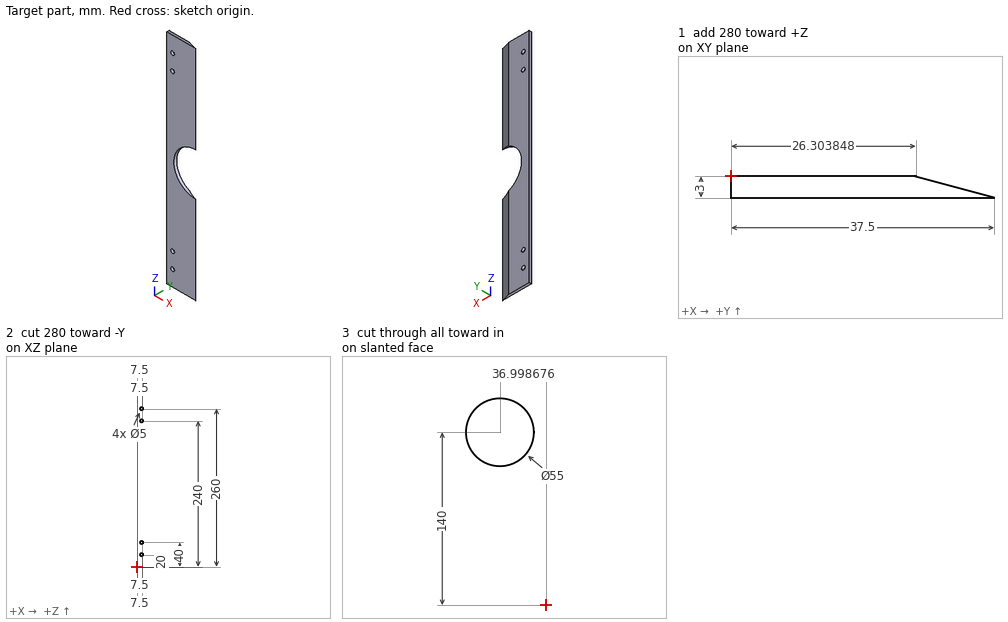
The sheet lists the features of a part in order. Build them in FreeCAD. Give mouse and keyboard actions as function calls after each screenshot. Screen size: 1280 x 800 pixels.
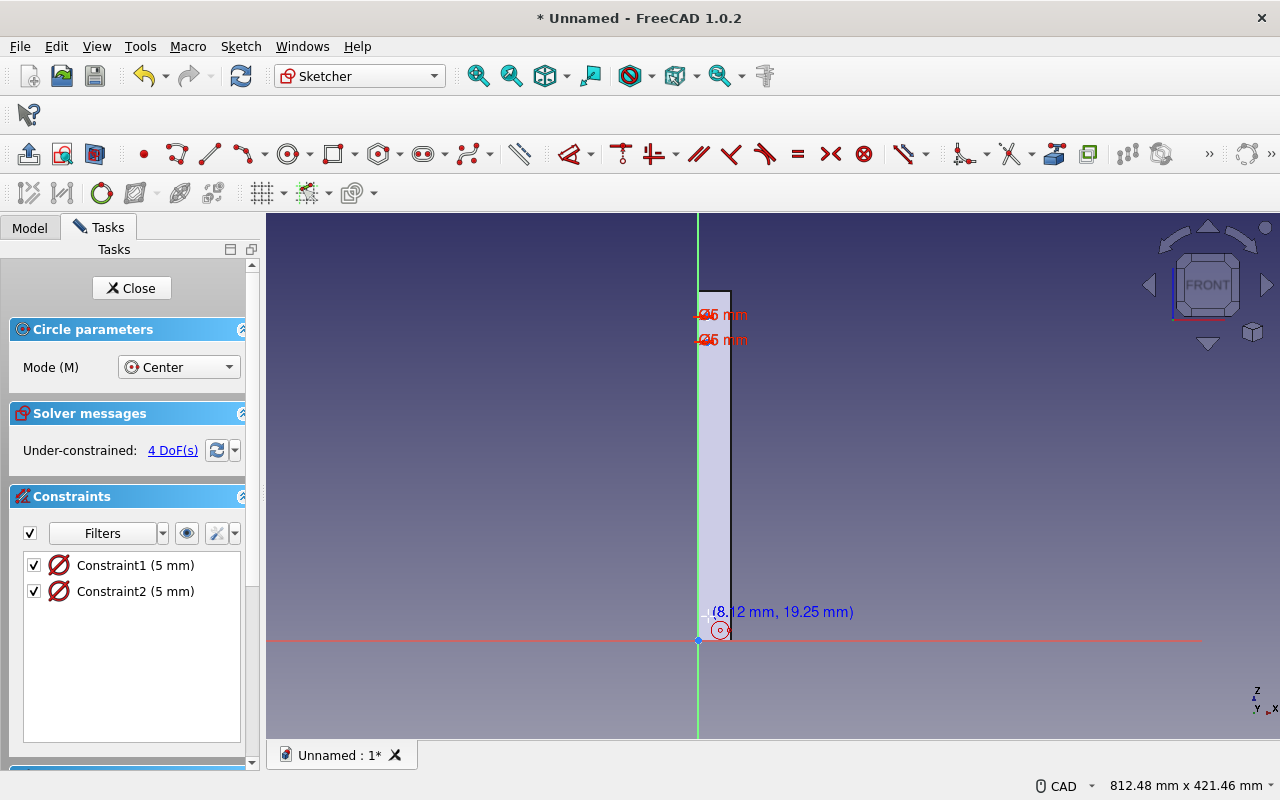
scroll(708, 616, up, 3)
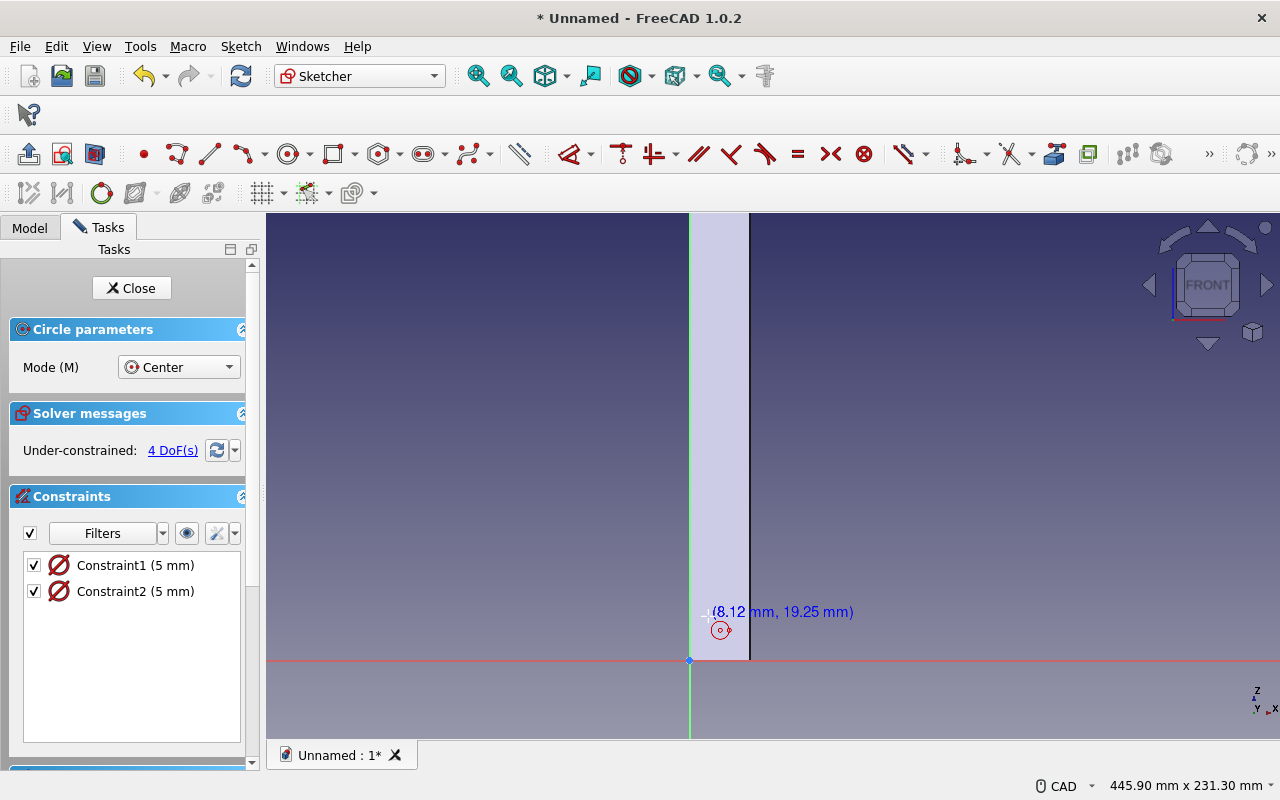
click(707, 615)
move(711, 611)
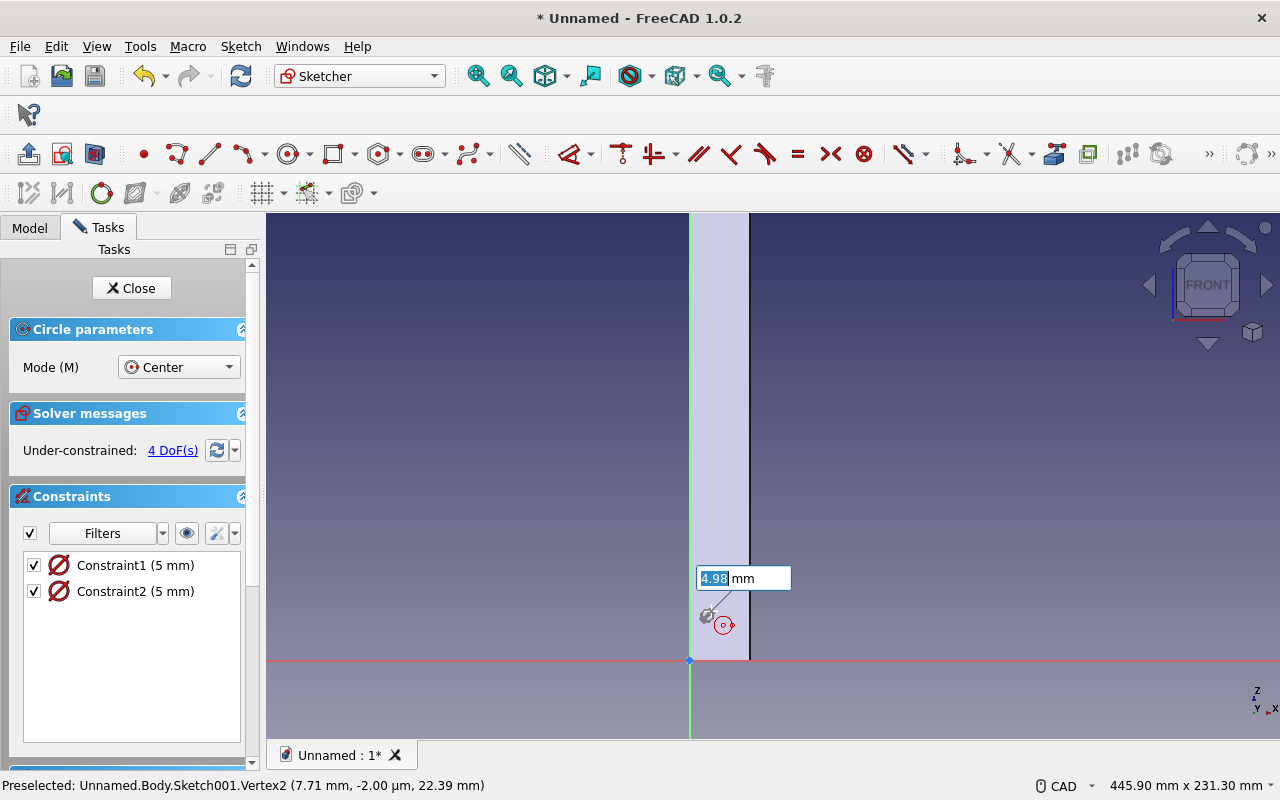
text(5)
key(Return)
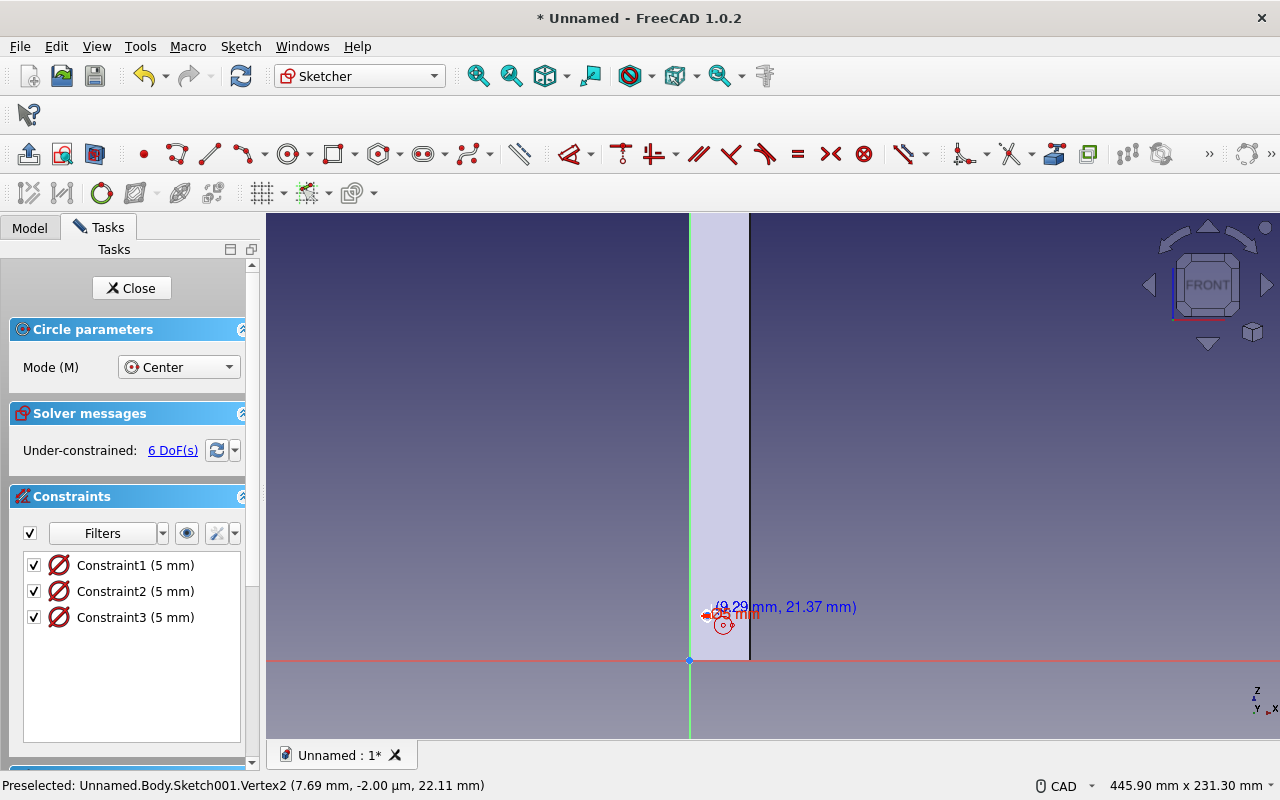
scroll(707, 570, up, 7)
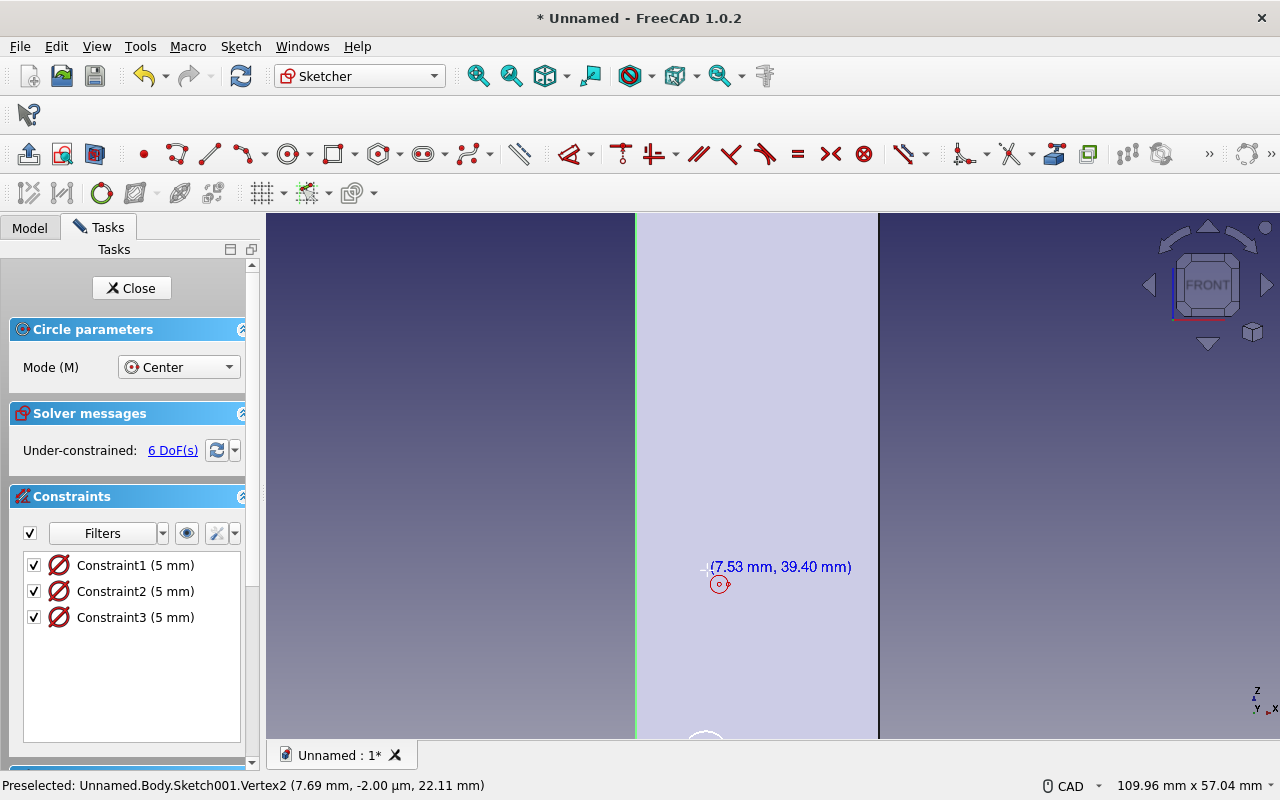
scroll(708, 594, down, 10)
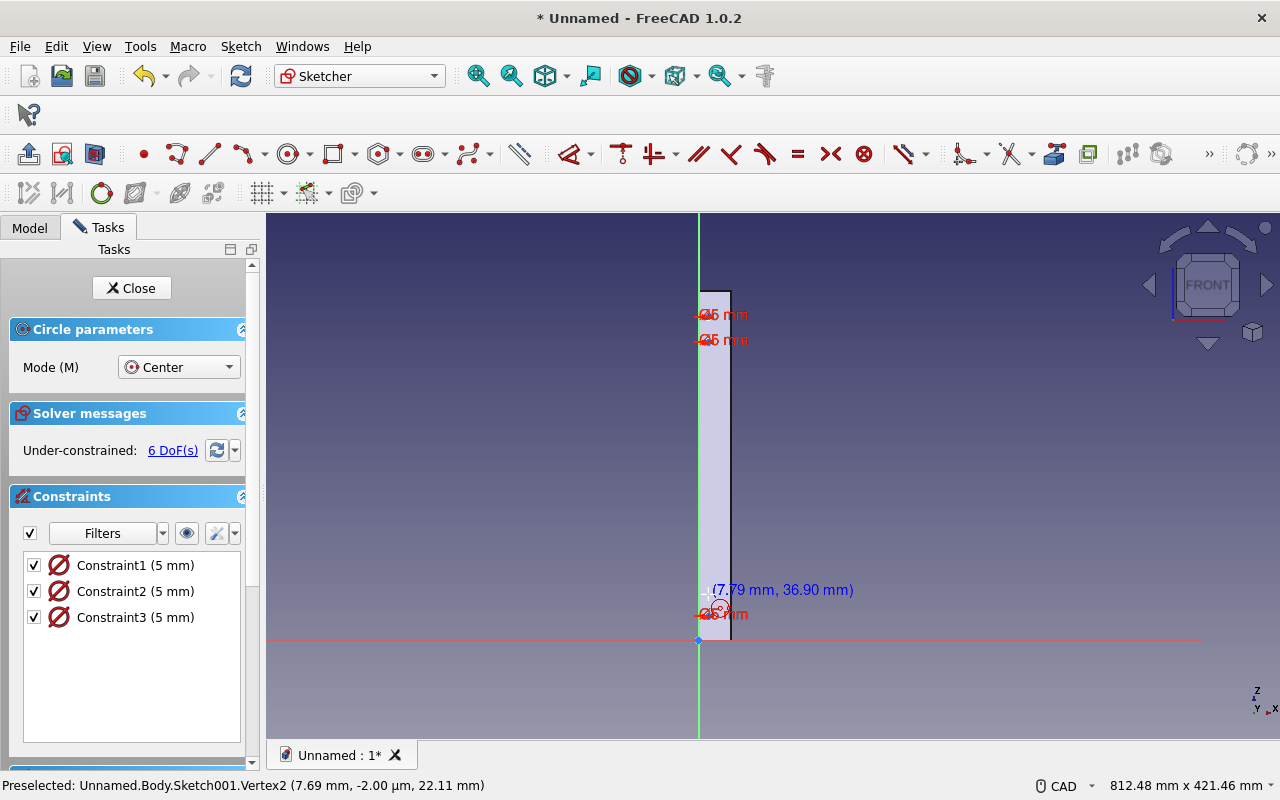
scroll(708, 591, up, 3)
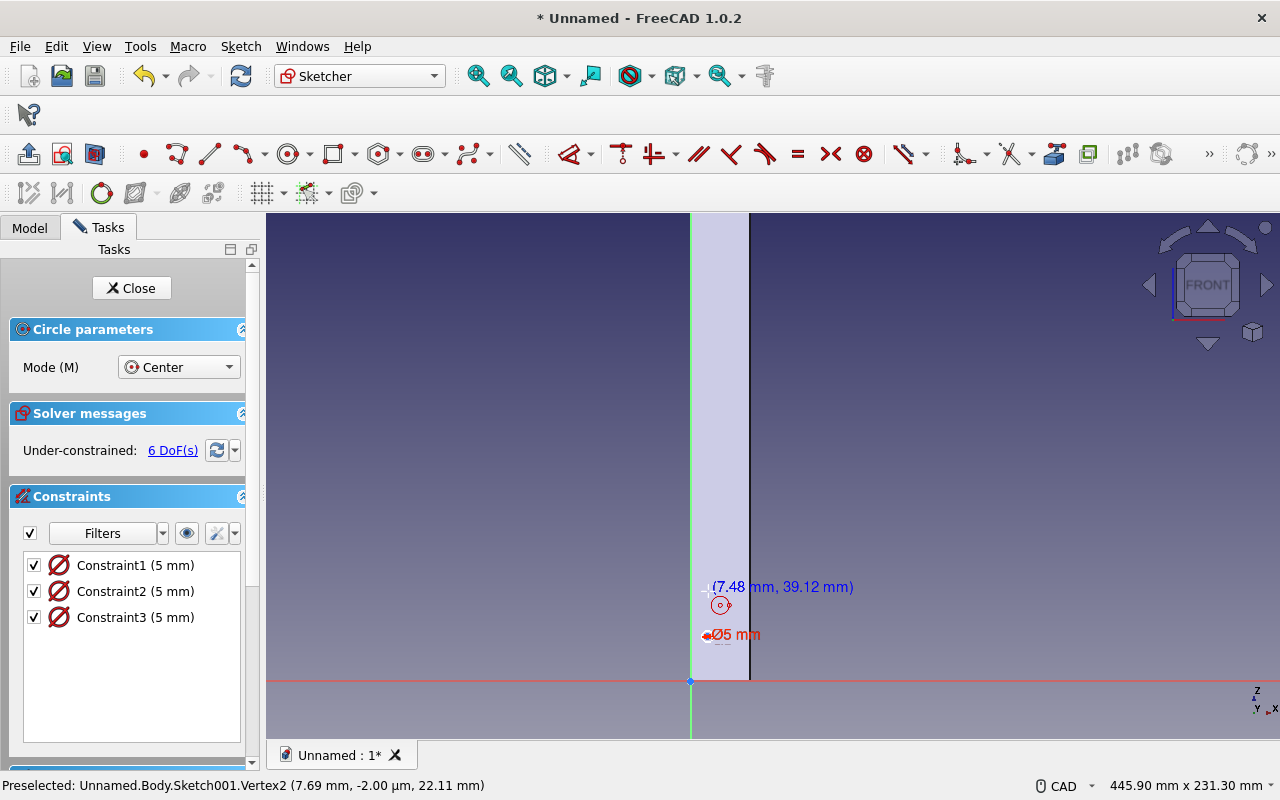
click(708, 590)
move(712, 586)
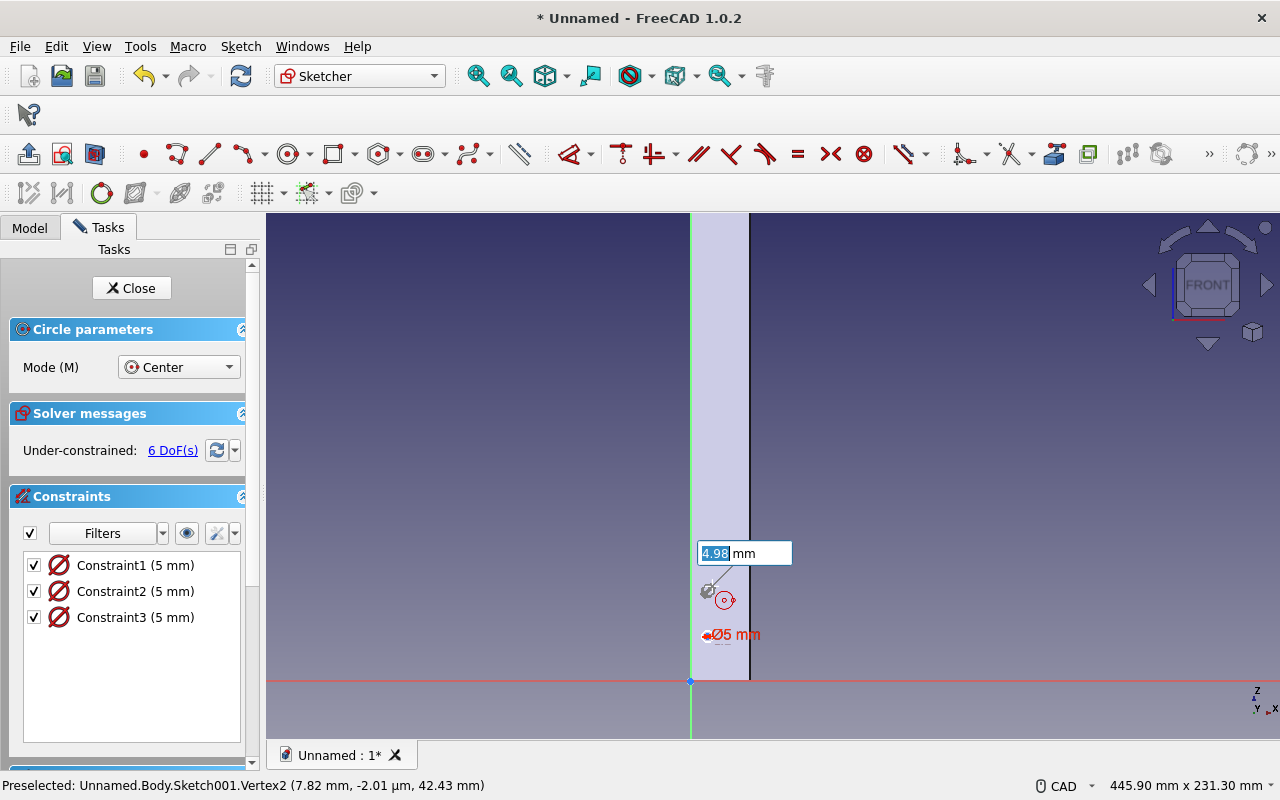
text(5)
key(Return)
key(Escape)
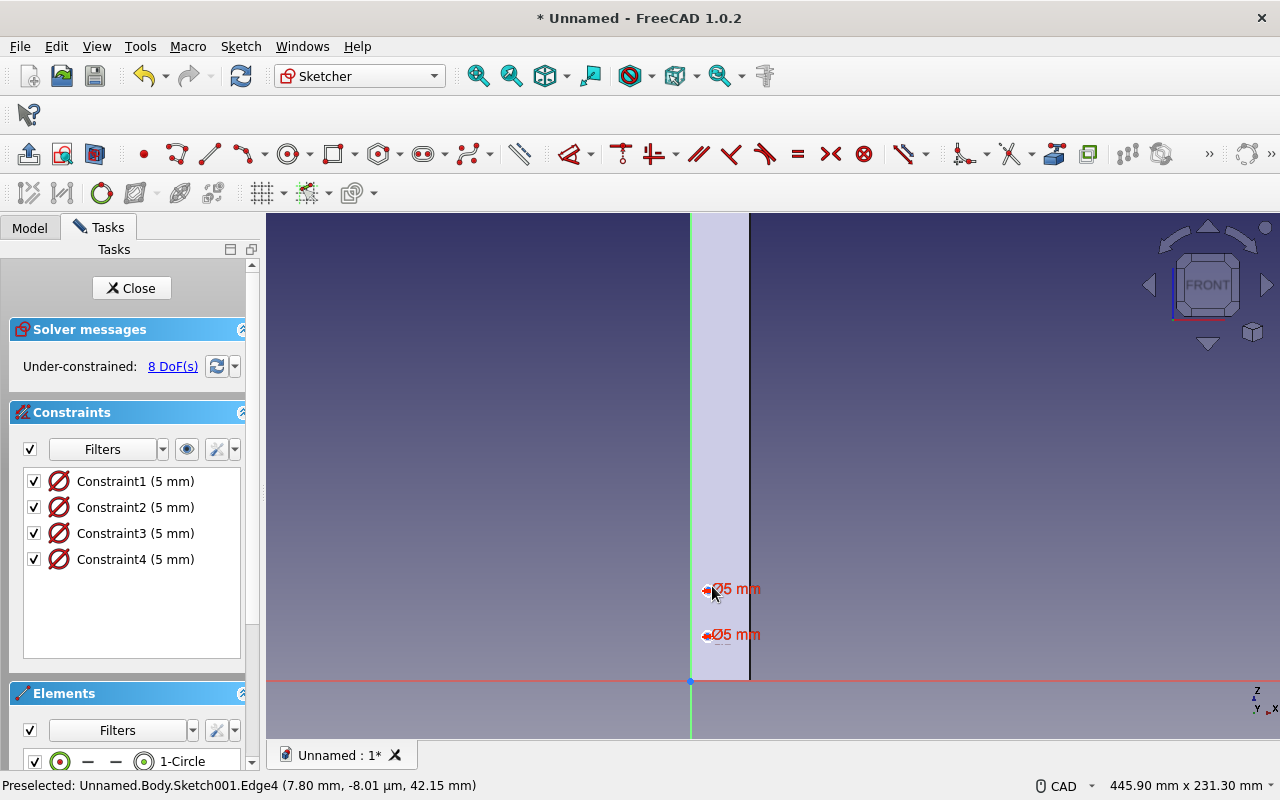
click(568, 154)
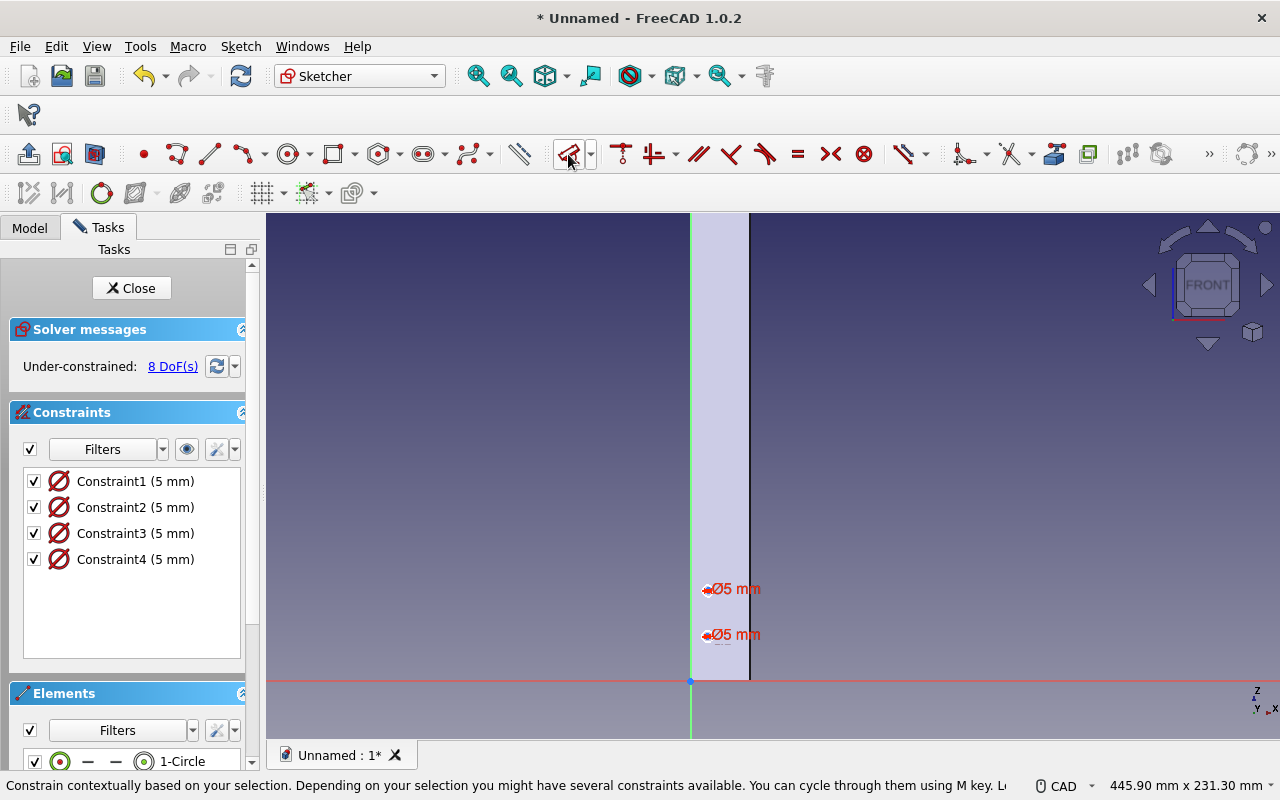
click(708, 637)
click(657, 659)